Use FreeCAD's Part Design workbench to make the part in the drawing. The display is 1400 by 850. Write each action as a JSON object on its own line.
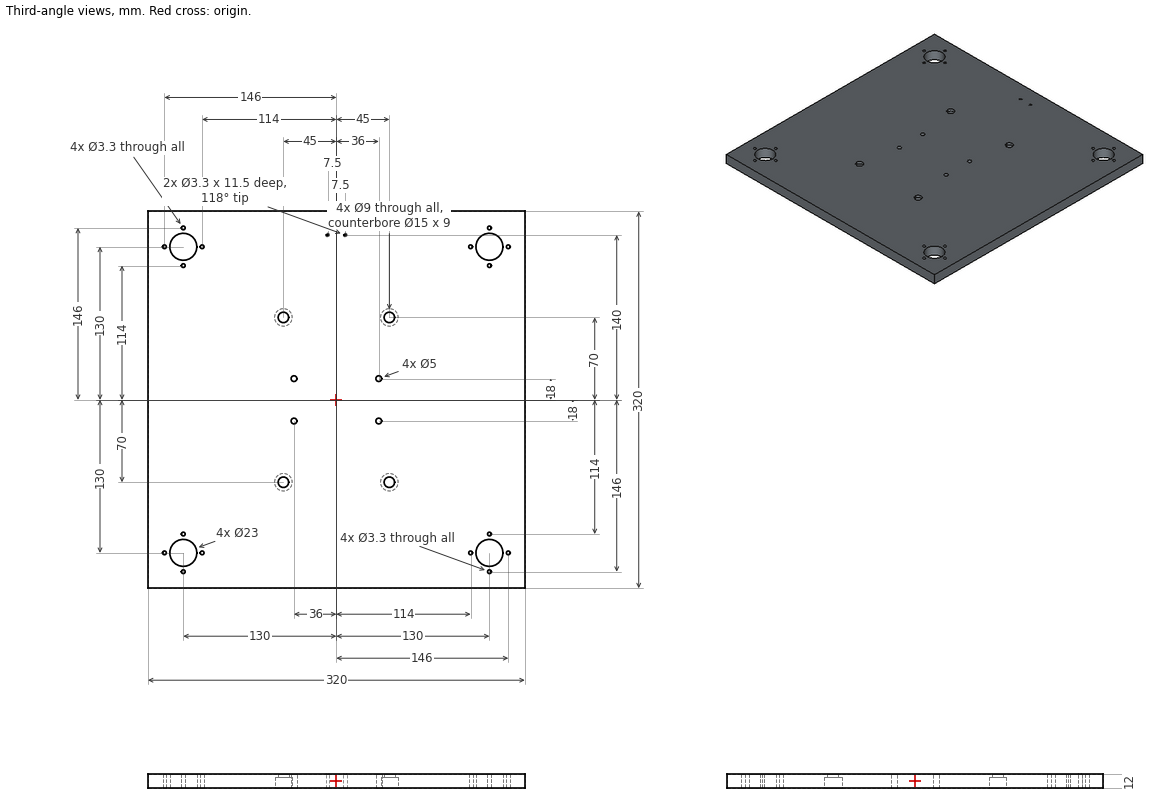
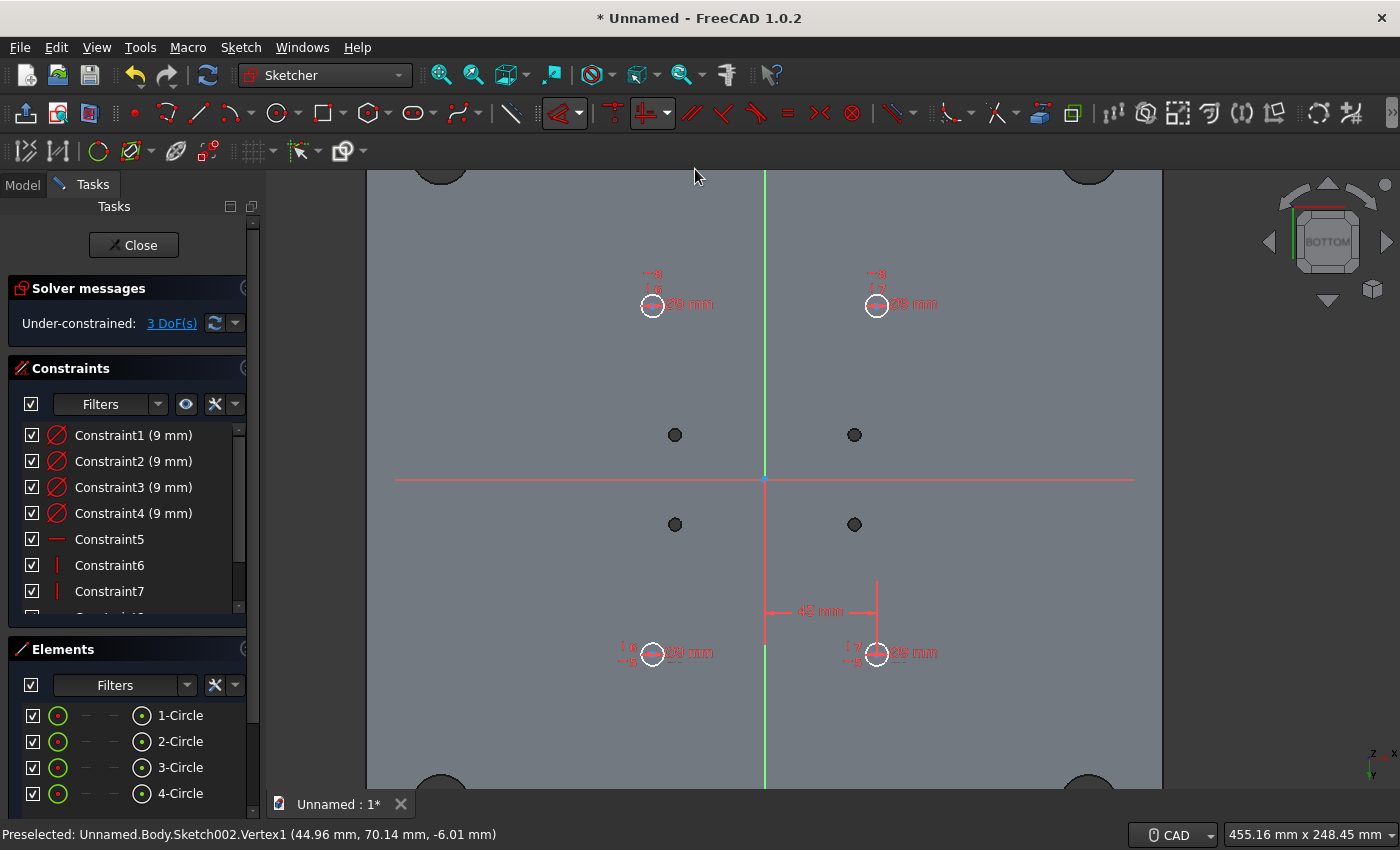
{"action": "left_click", "coordinate": [877, 655]}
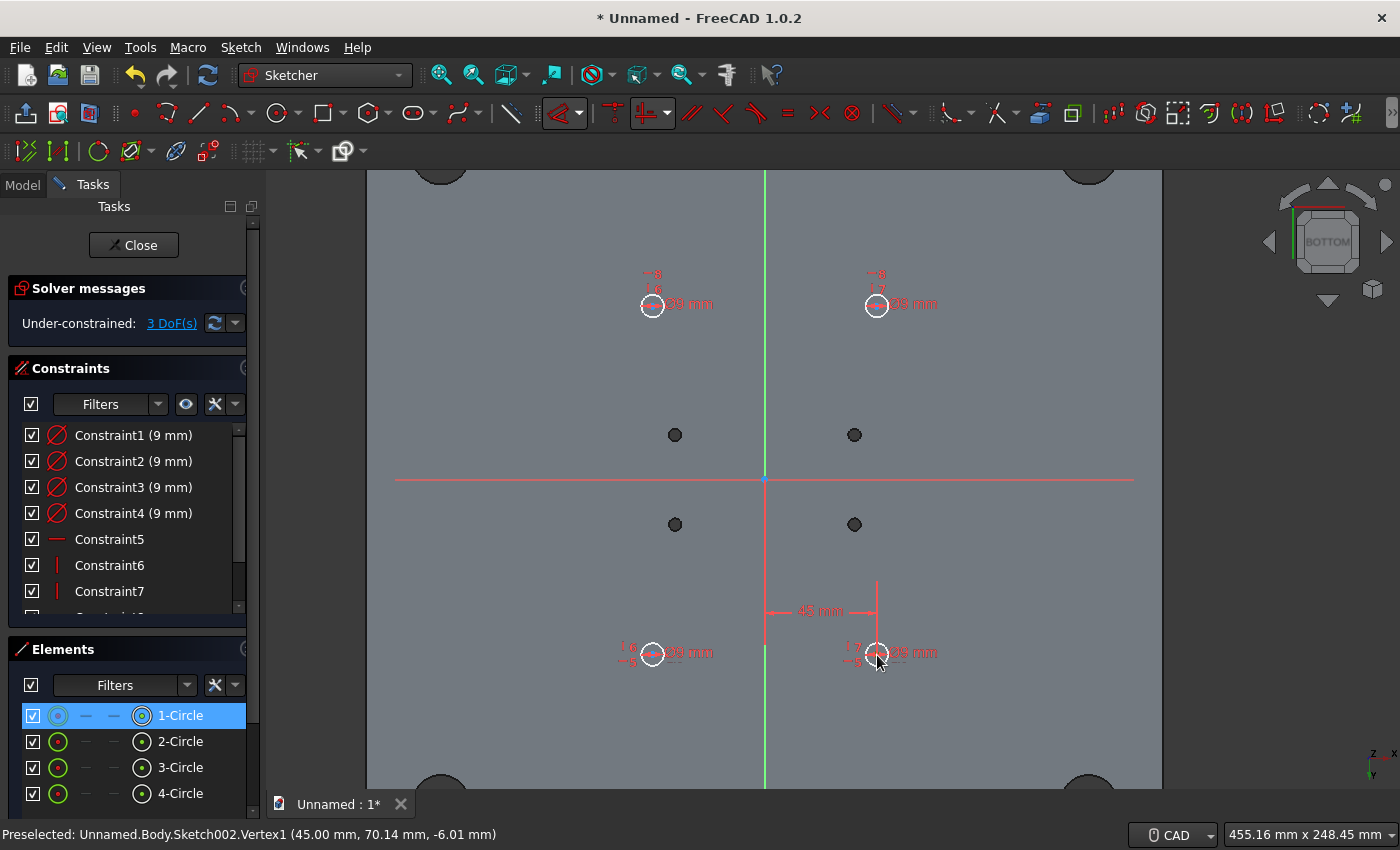
{"action": "key", "text": "i"}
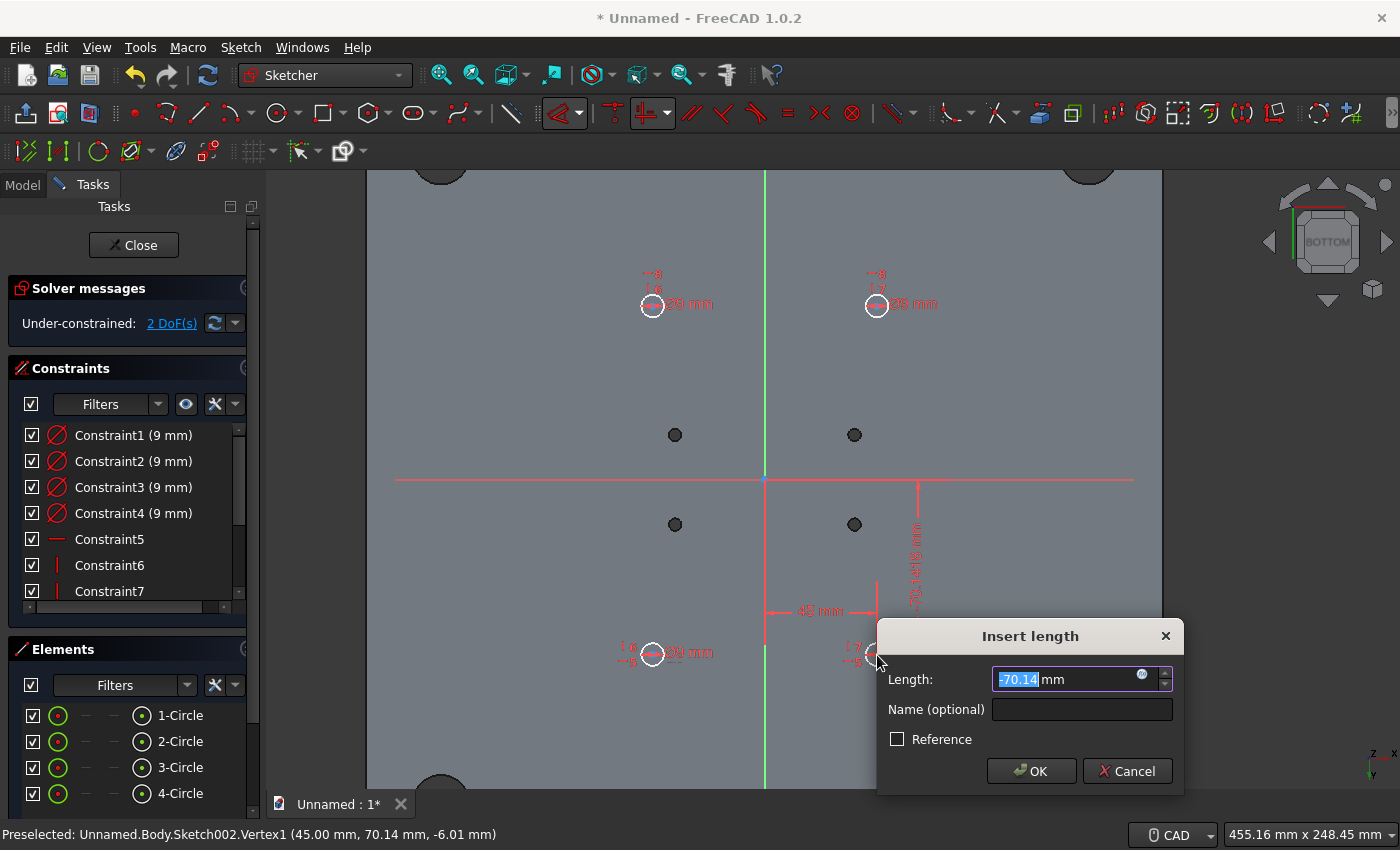
{"action": "type", "text": "-70"}
{"action": "key", "text": "Return"}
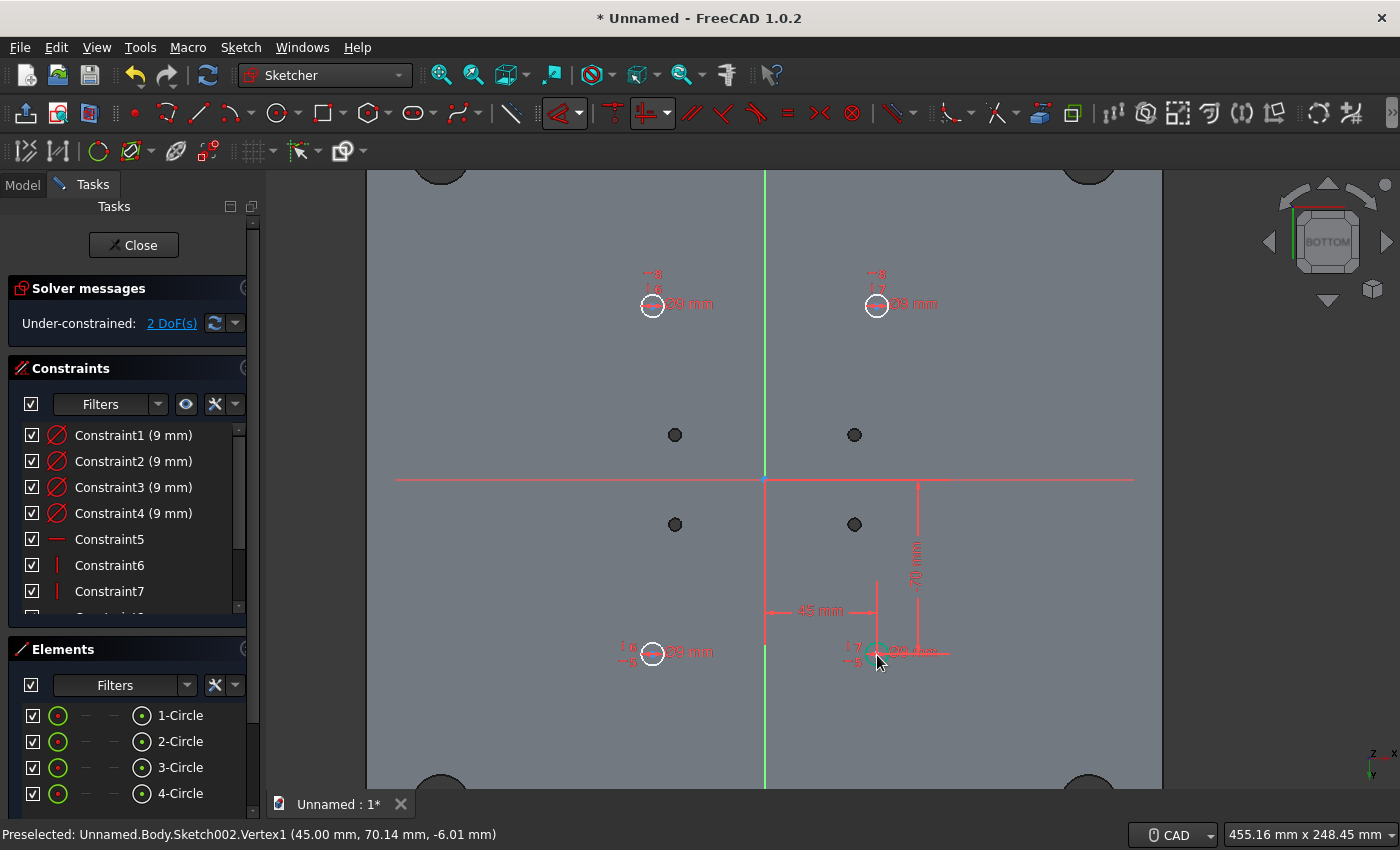
{"action": "left_click", "coordinate": [653, 654]}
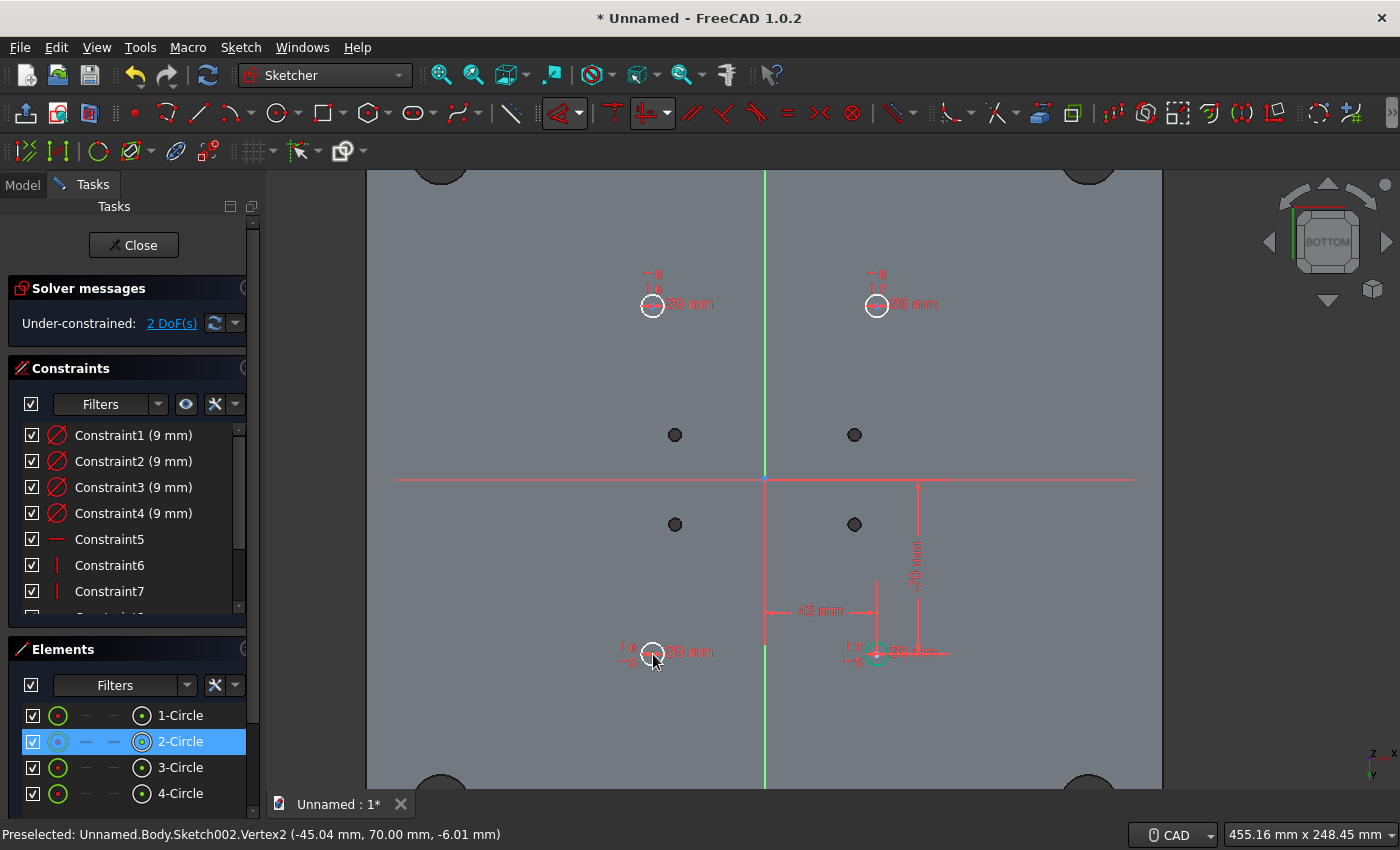
{"action": "key", "text": "l"}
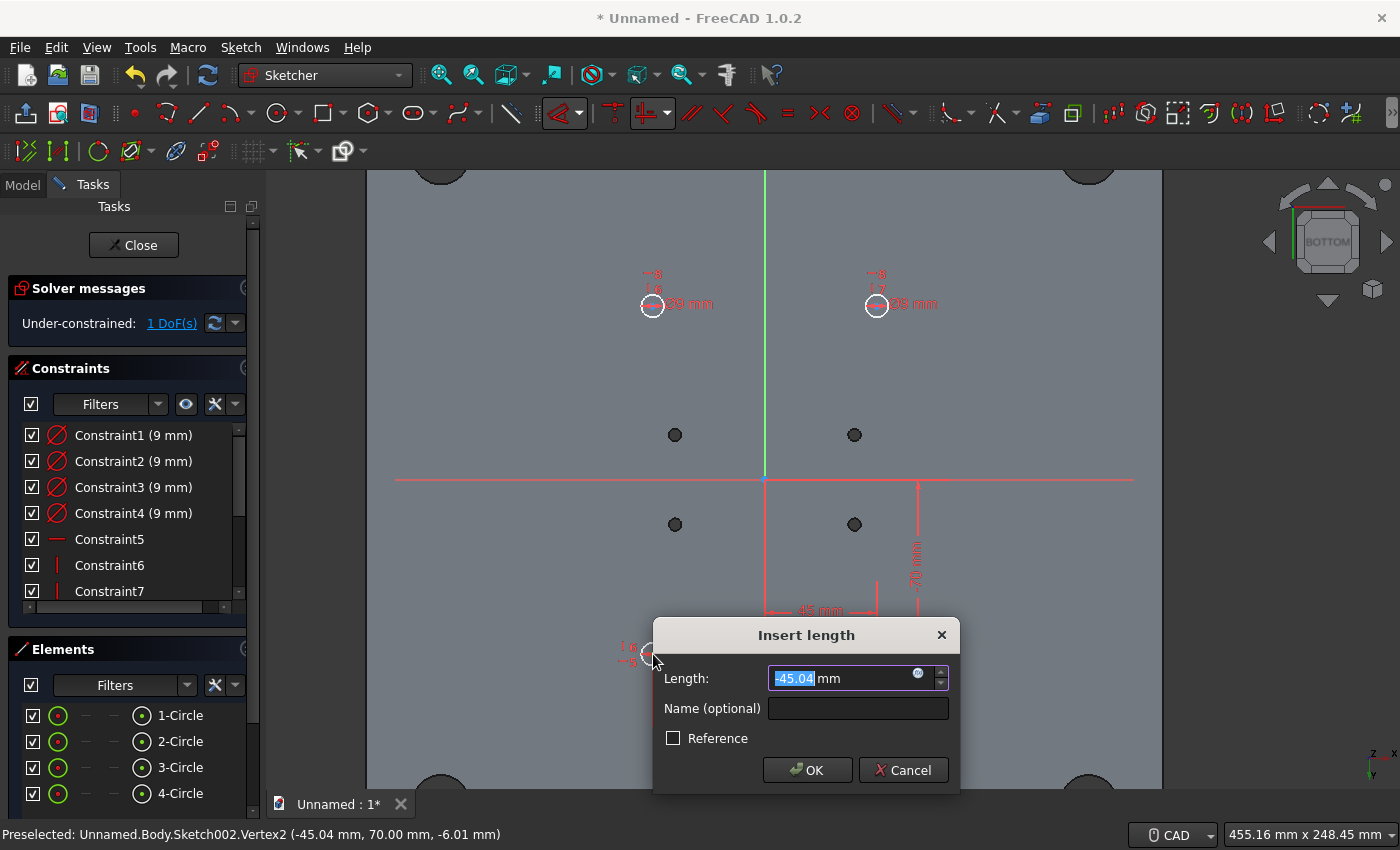
{"action": "type", "text": "-45"}
{"action": "key", "text": "Return"}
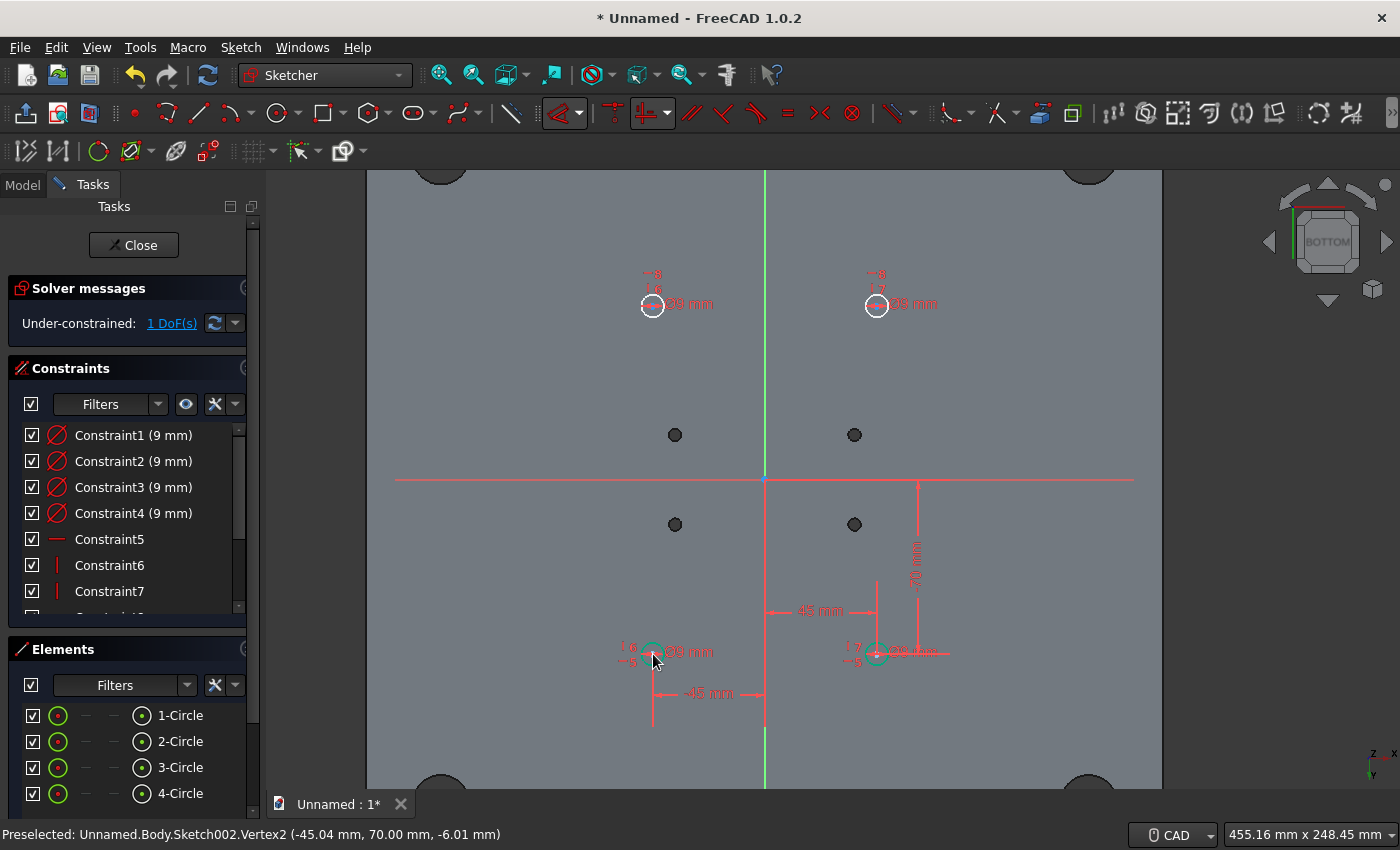
{"action": "left_click", "coordinate": [653, 306]}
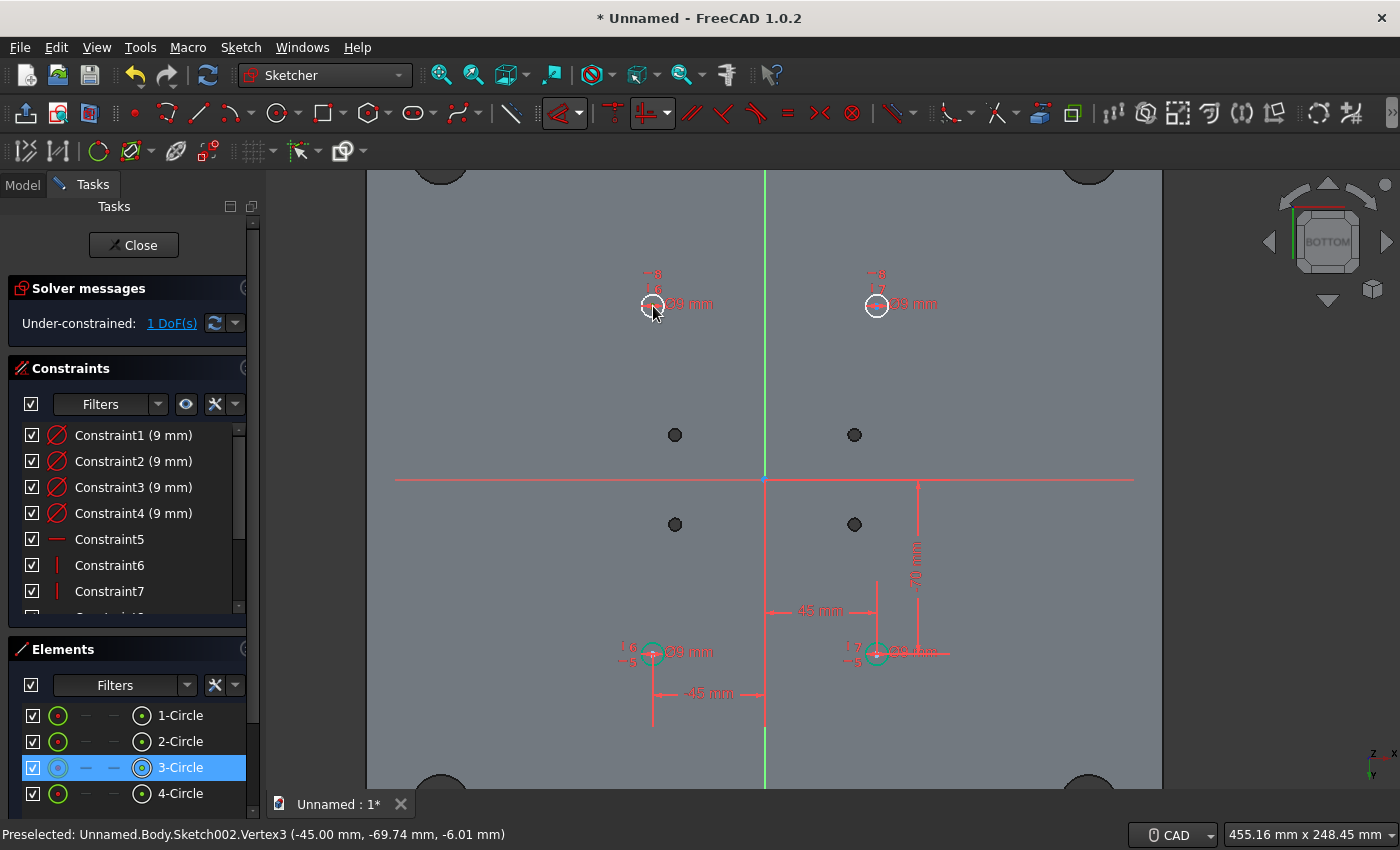
{"action": "left_click", "coordinate": [582, 114]}